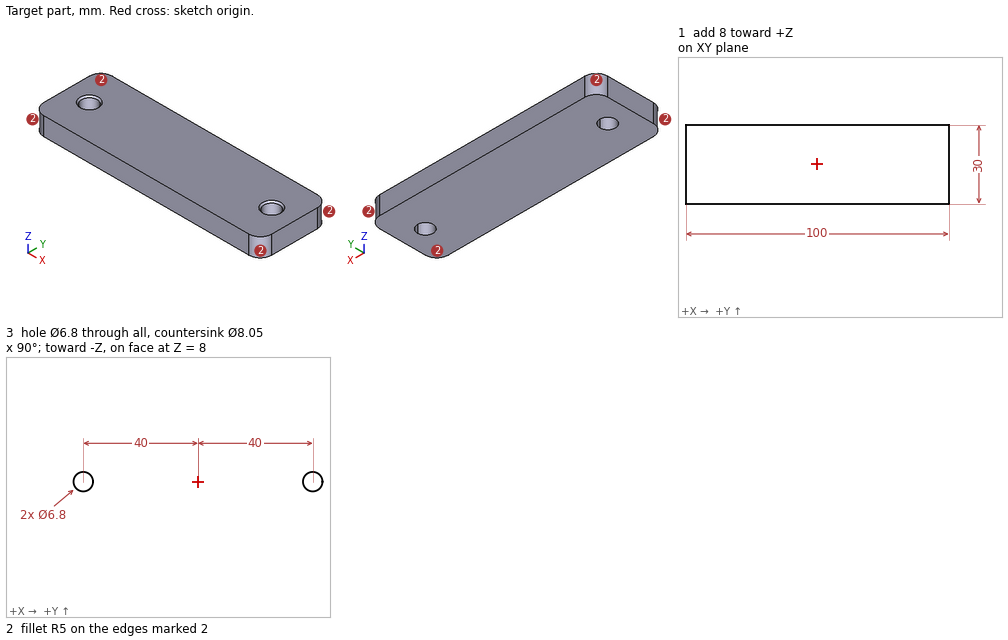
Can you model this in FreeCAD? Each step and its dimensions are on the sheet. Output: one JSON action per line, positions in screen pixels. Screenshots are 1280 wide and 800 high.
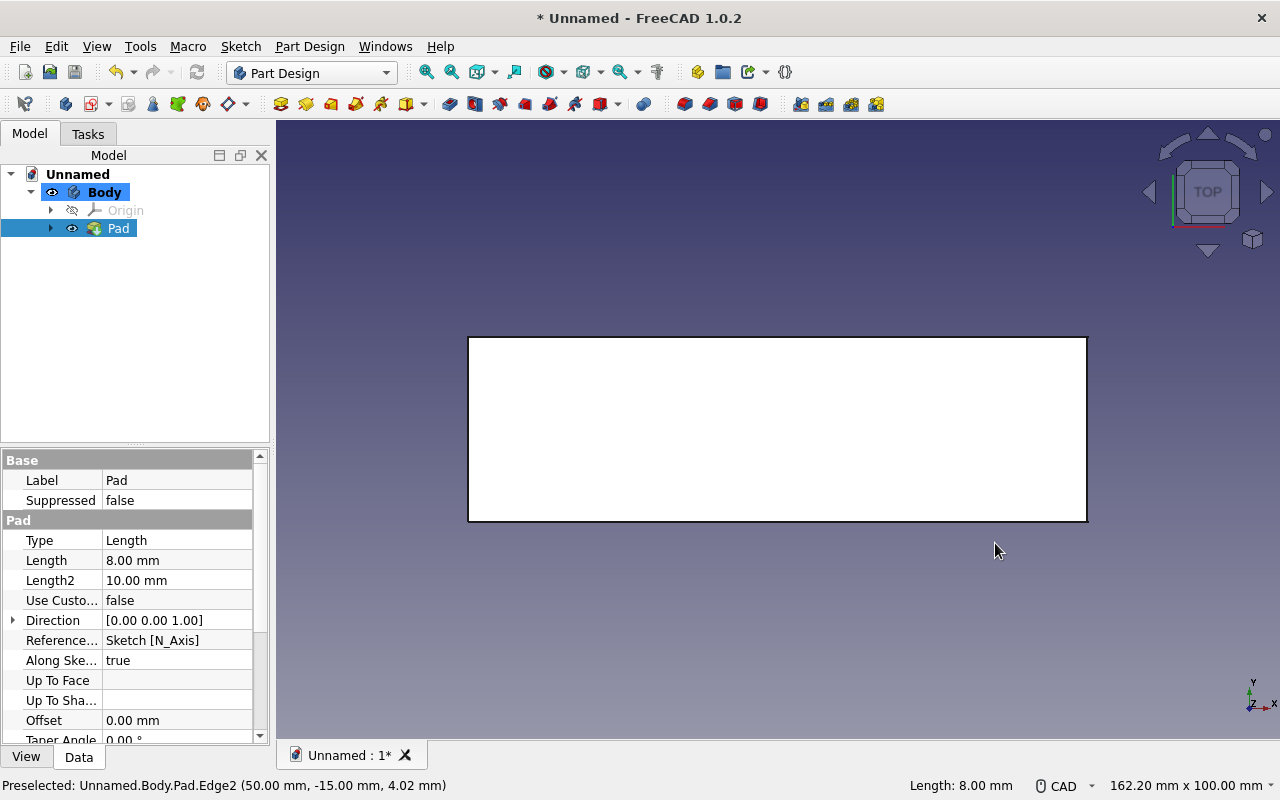
{"action": "key", "text": "1"}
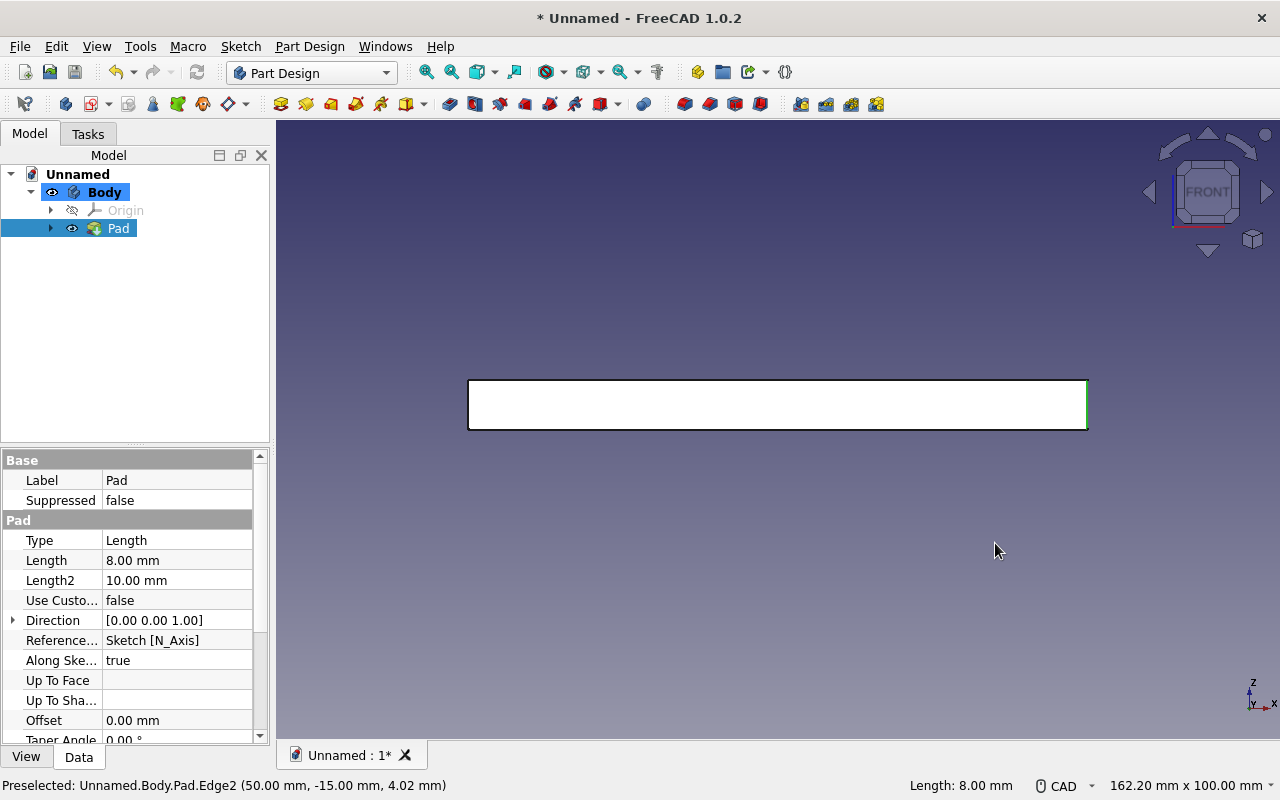
{"action": "left_click", "coordinate": [468, 404], "text": "ctrl"}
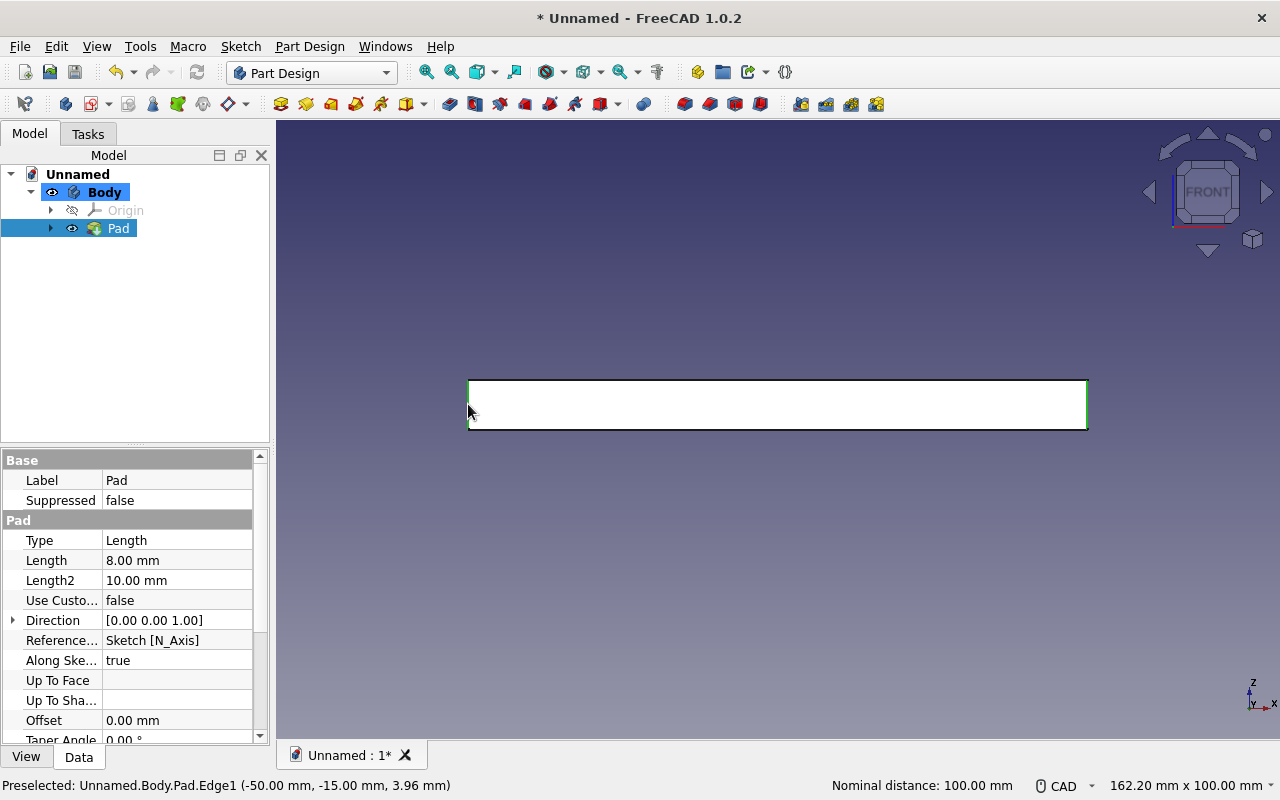
{"action": "key", "text": "3"}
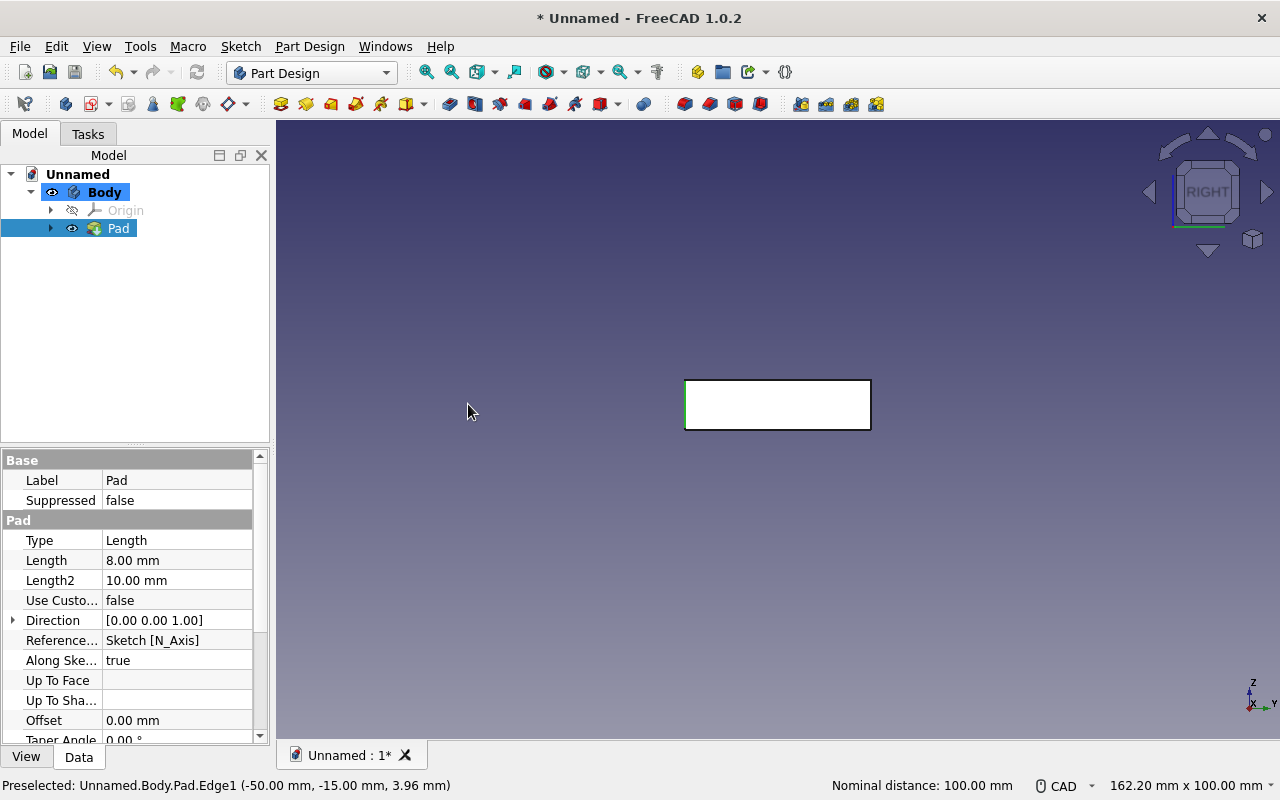
{"action": "left_click", "coordinate": [427, 72]}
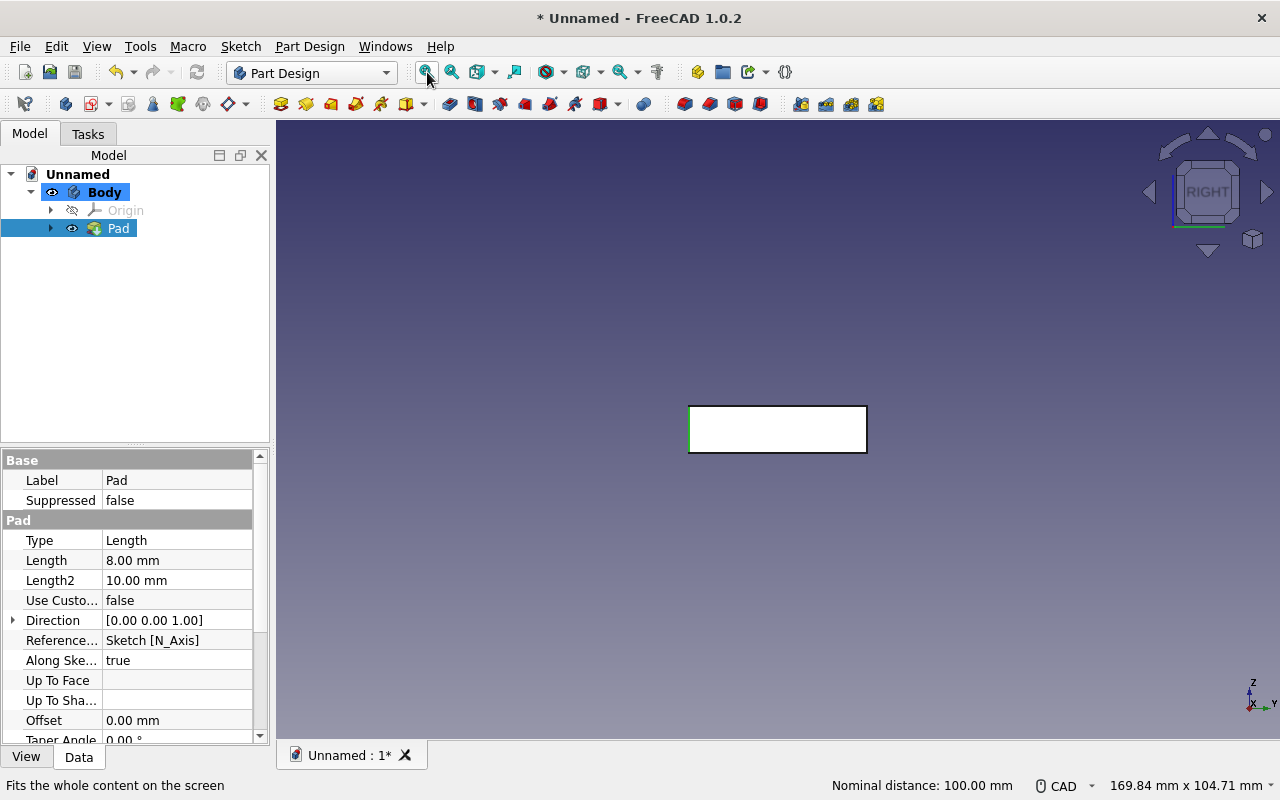
{"action": "left_click", "coordinate": [867, 428], "text": "ctrl"}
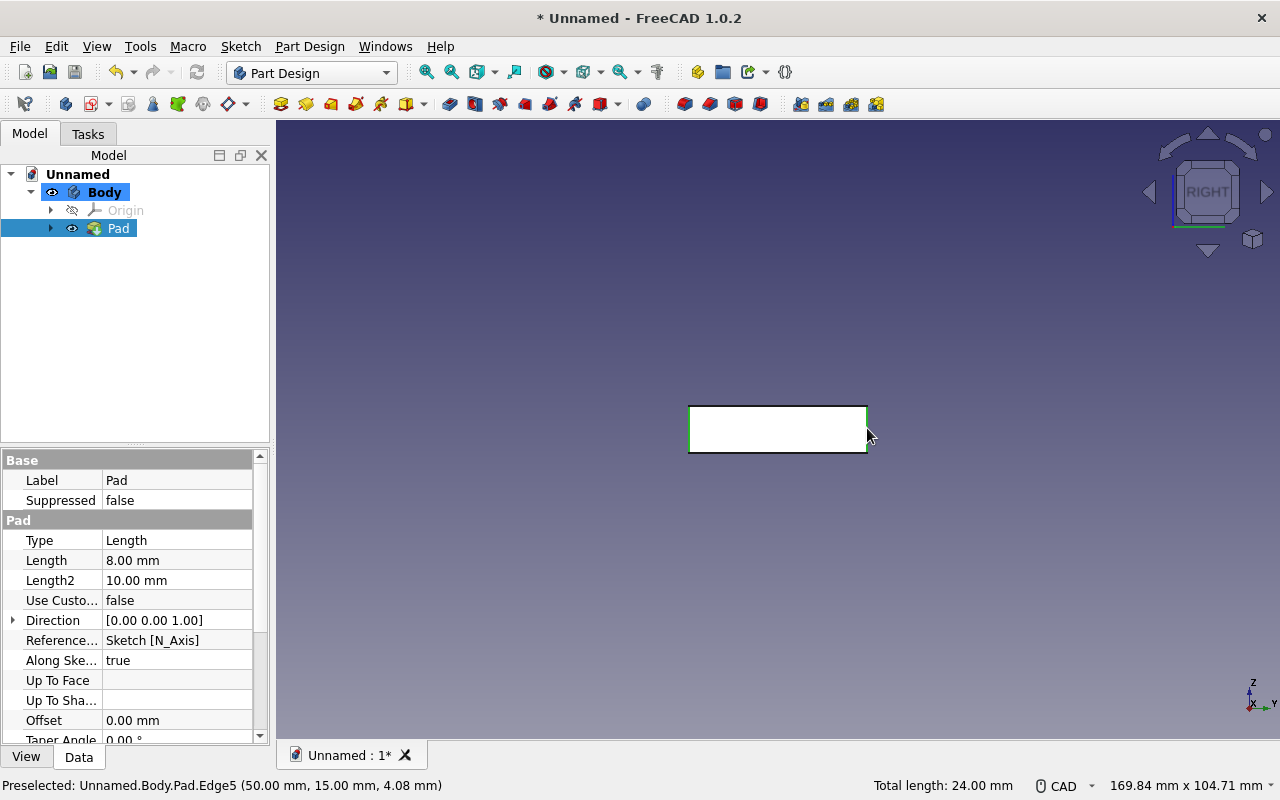
{"action": "key", "text": "5"}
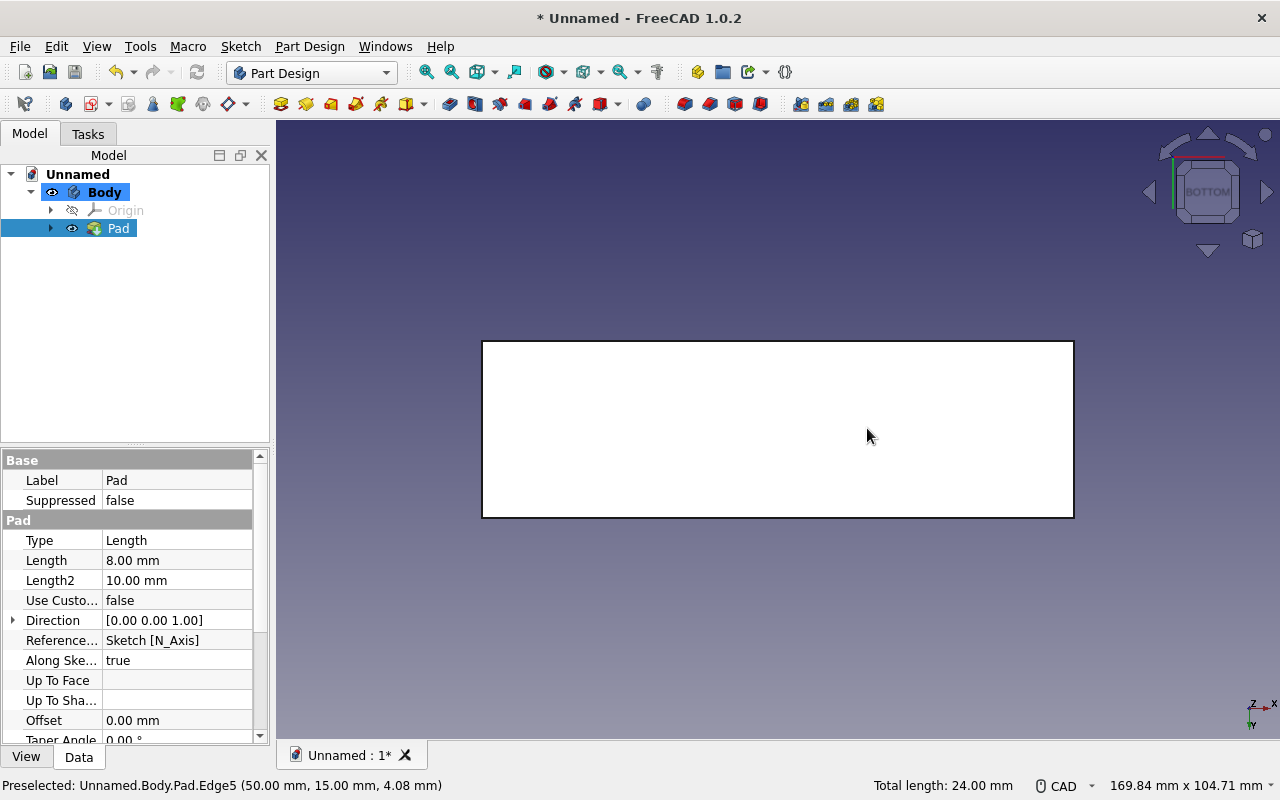
{"action": "key", "text": "4"}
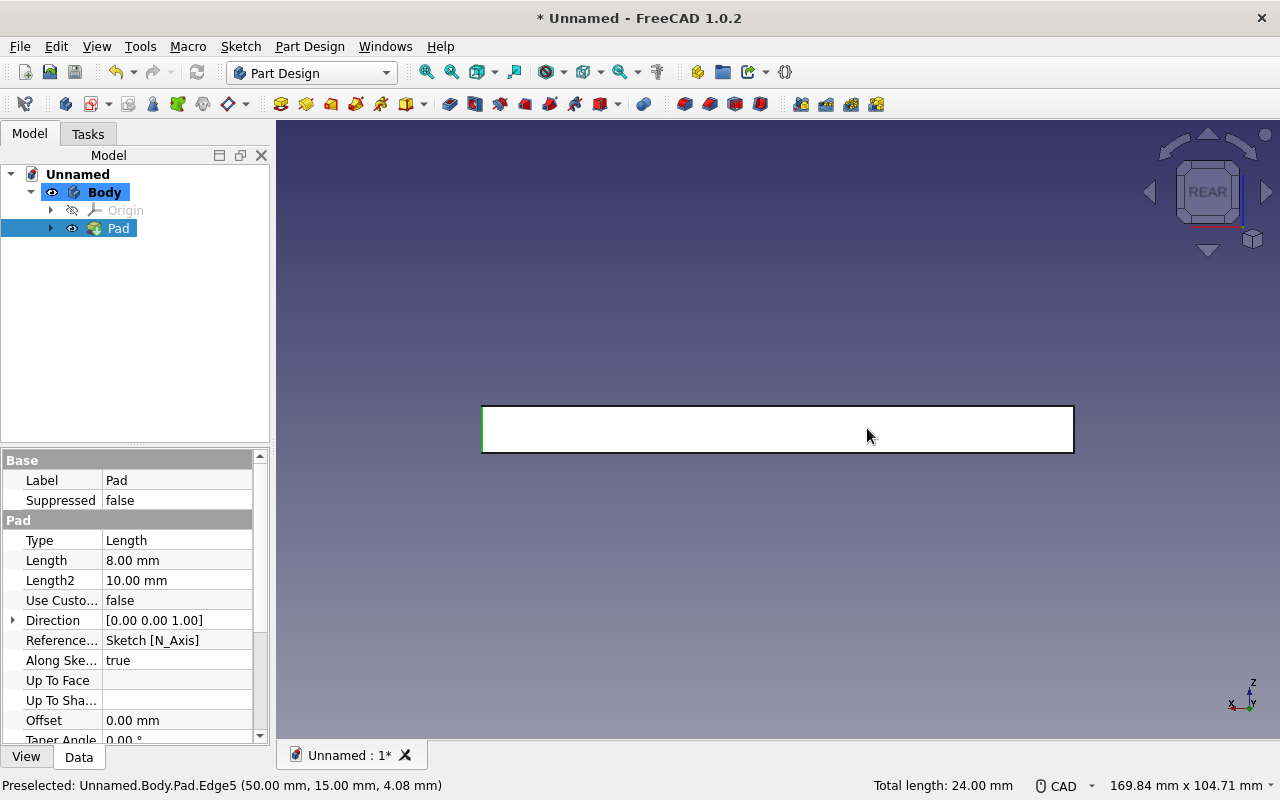
{"action": "left_click", "coordinate": [1074, 429], "text": "ctrl"}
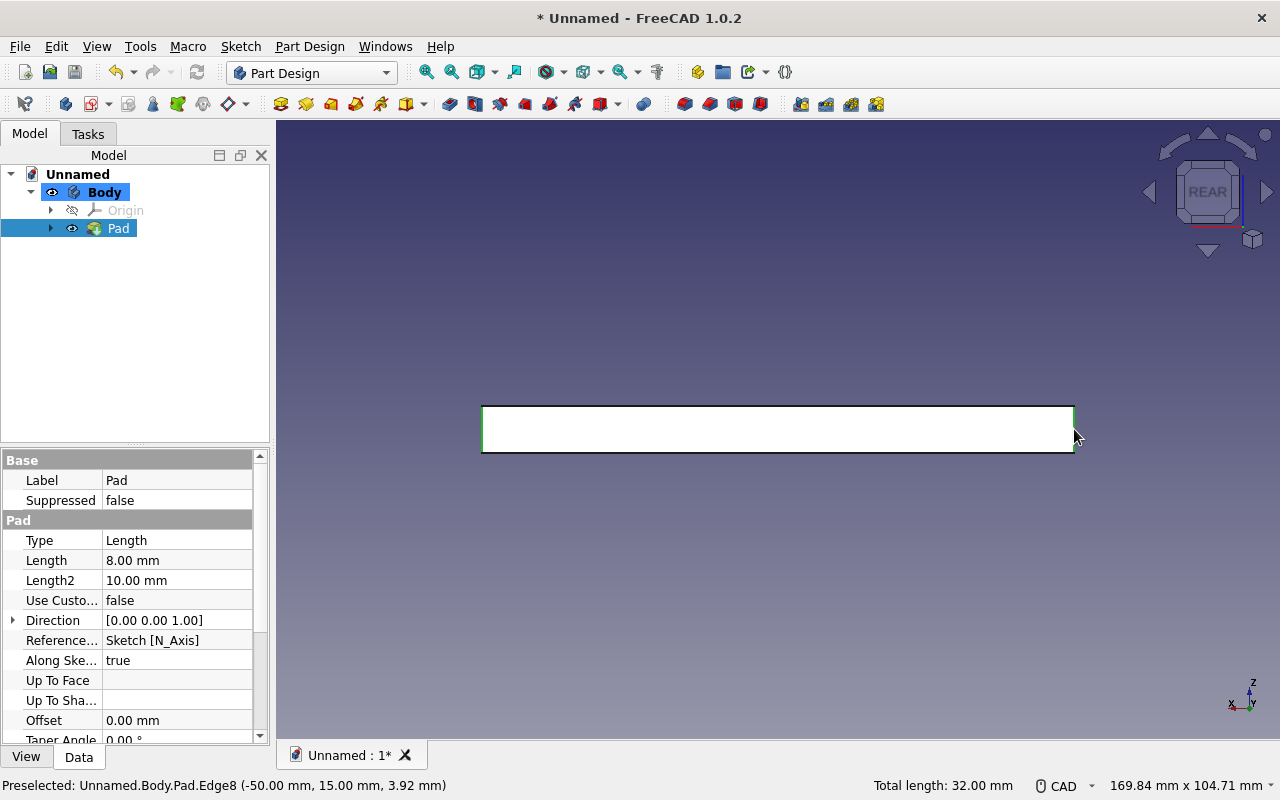
{"action": "left_click", "coordinate": [685, 104]}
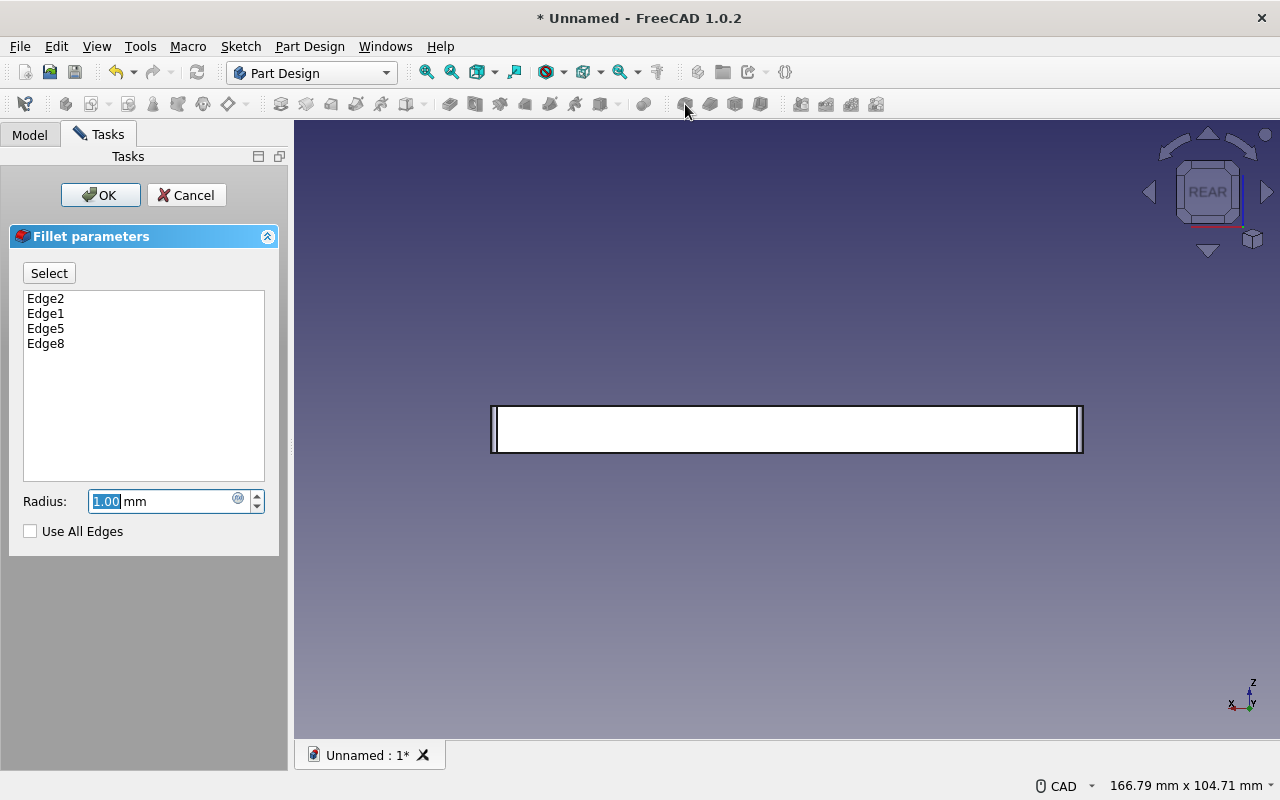
{"action": "type", "text": "5"}
{"action": "key", "text": "Tab"}